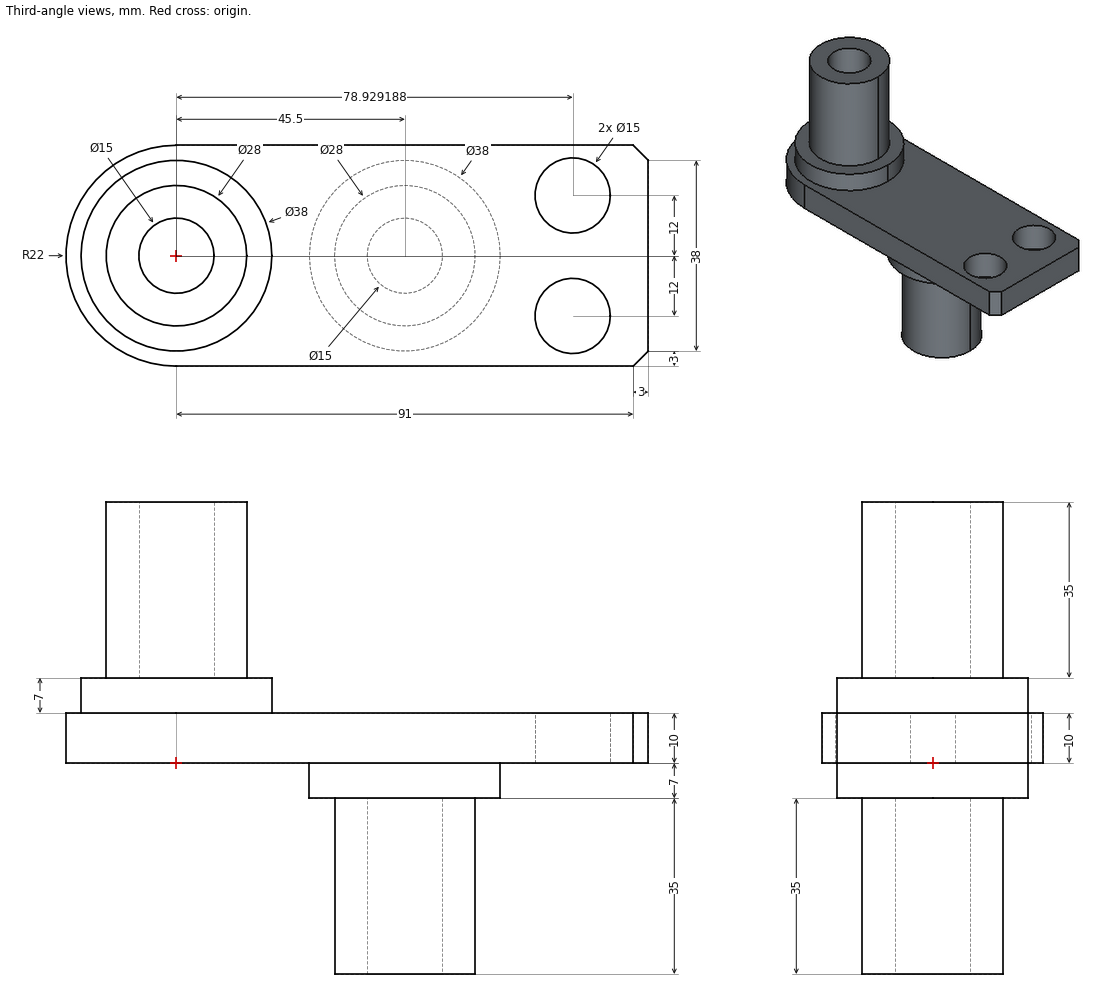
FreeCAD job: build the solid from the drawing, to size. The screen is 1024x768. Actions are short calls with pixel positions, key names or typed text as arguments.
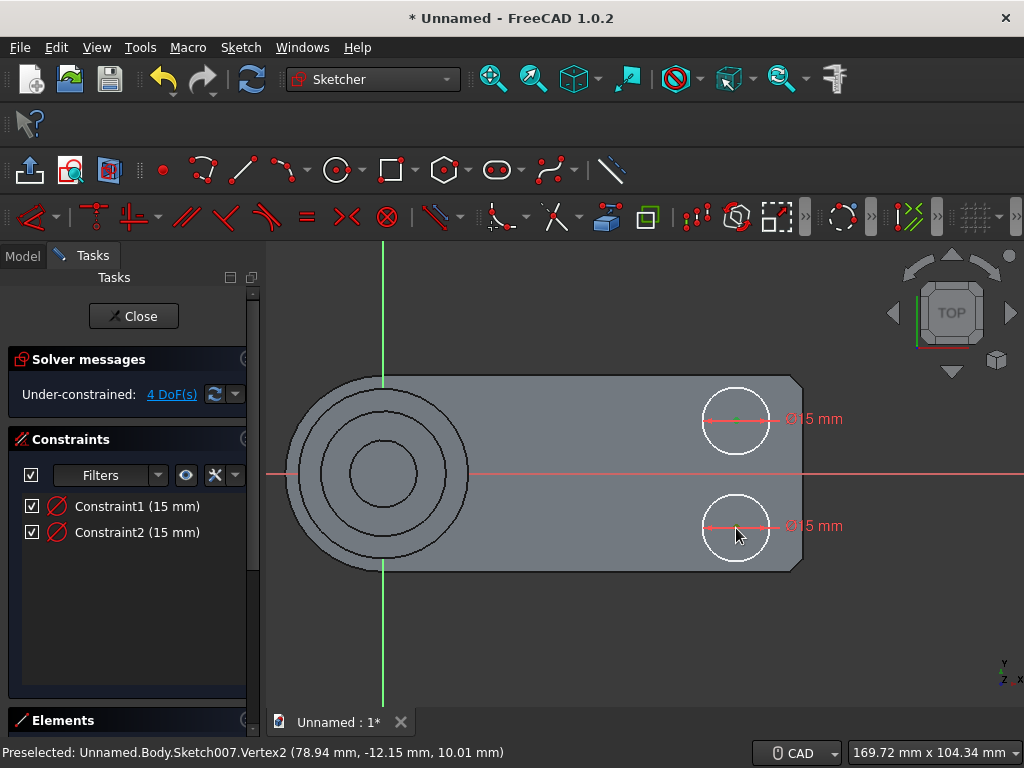
click(160, 218)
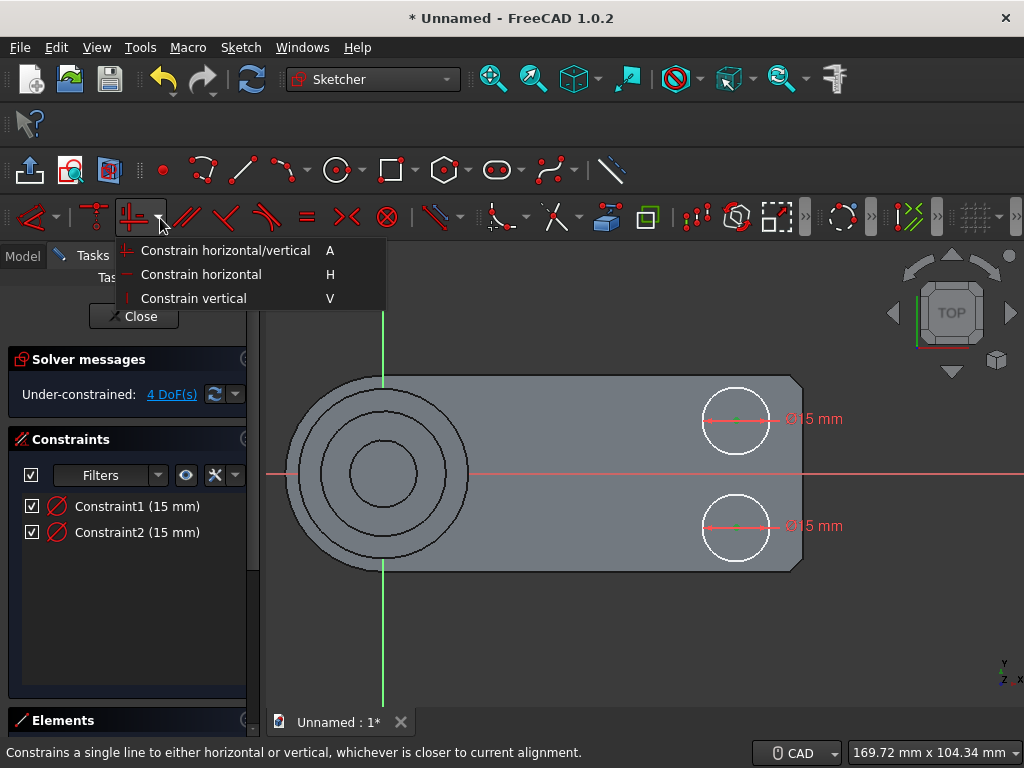
click(251, 298)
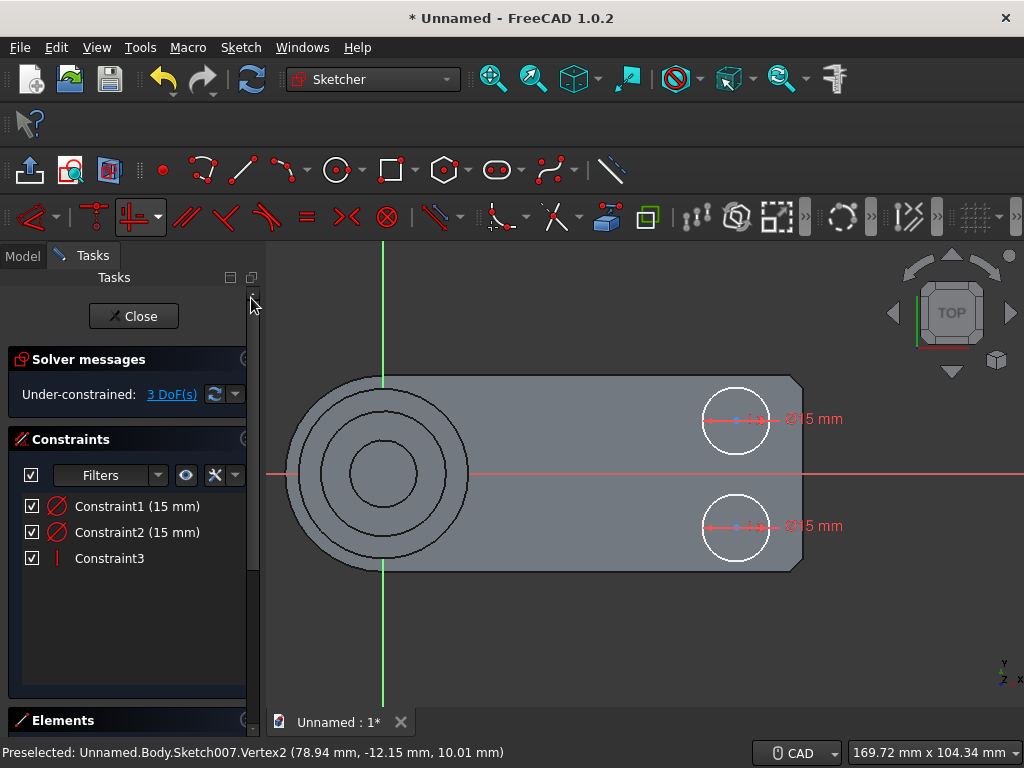
click(32, 218)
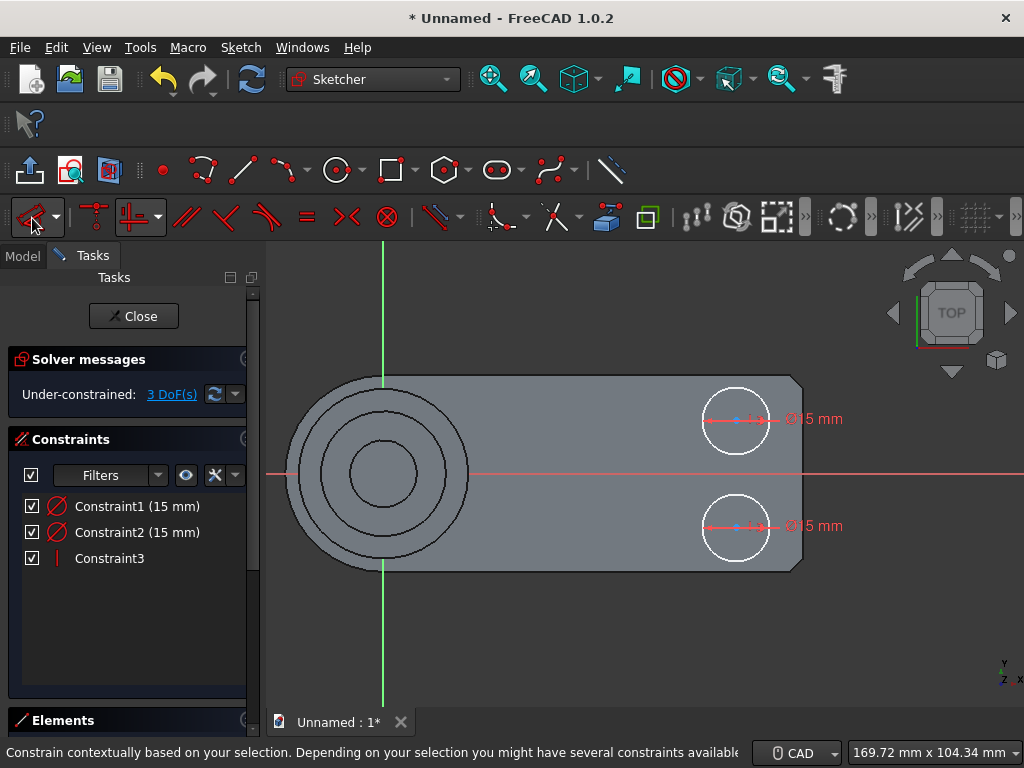
click(736, 421)
click(349, 447)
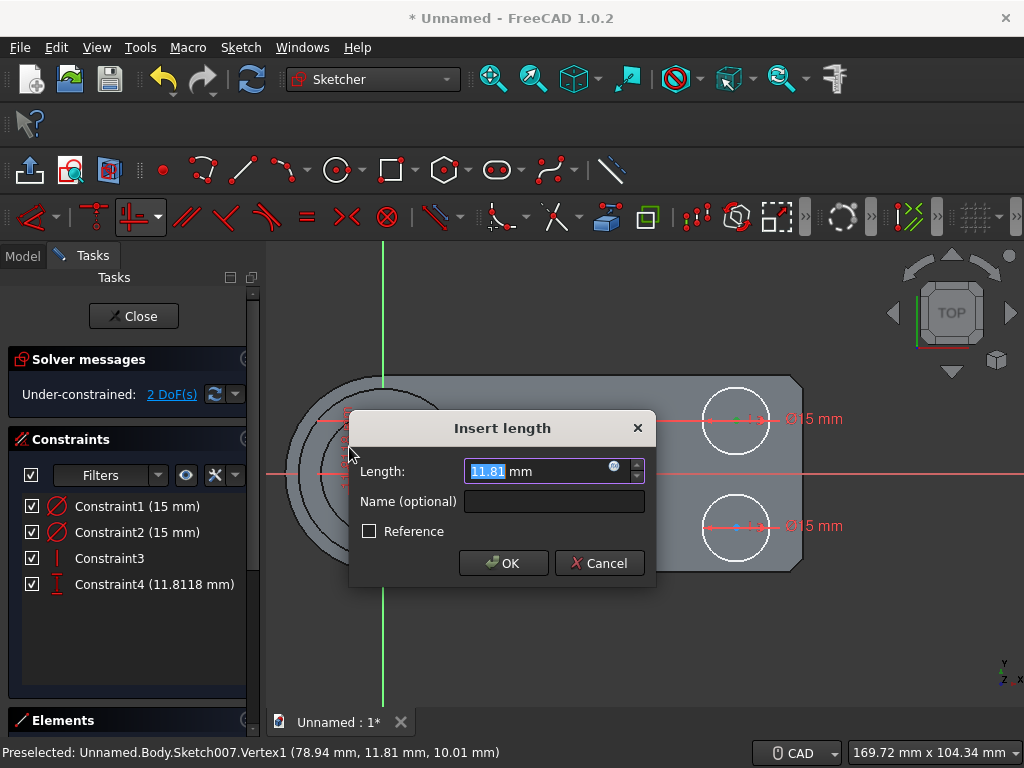
text(12)
key(Return)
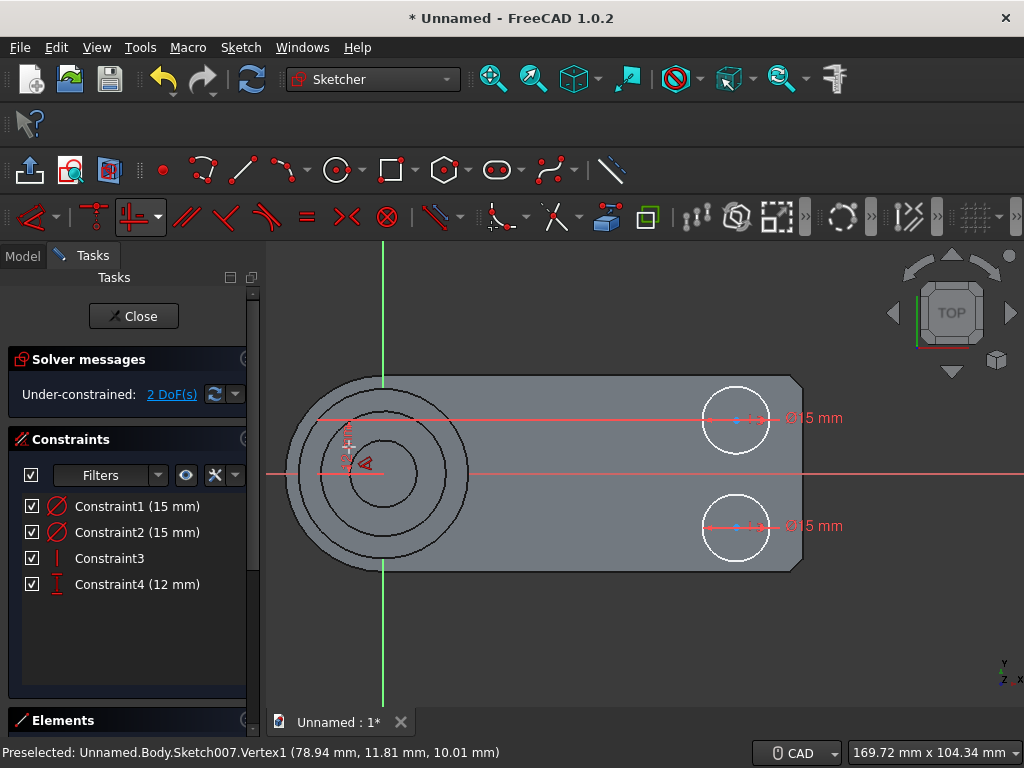
click(736, 528)
click(349, 501)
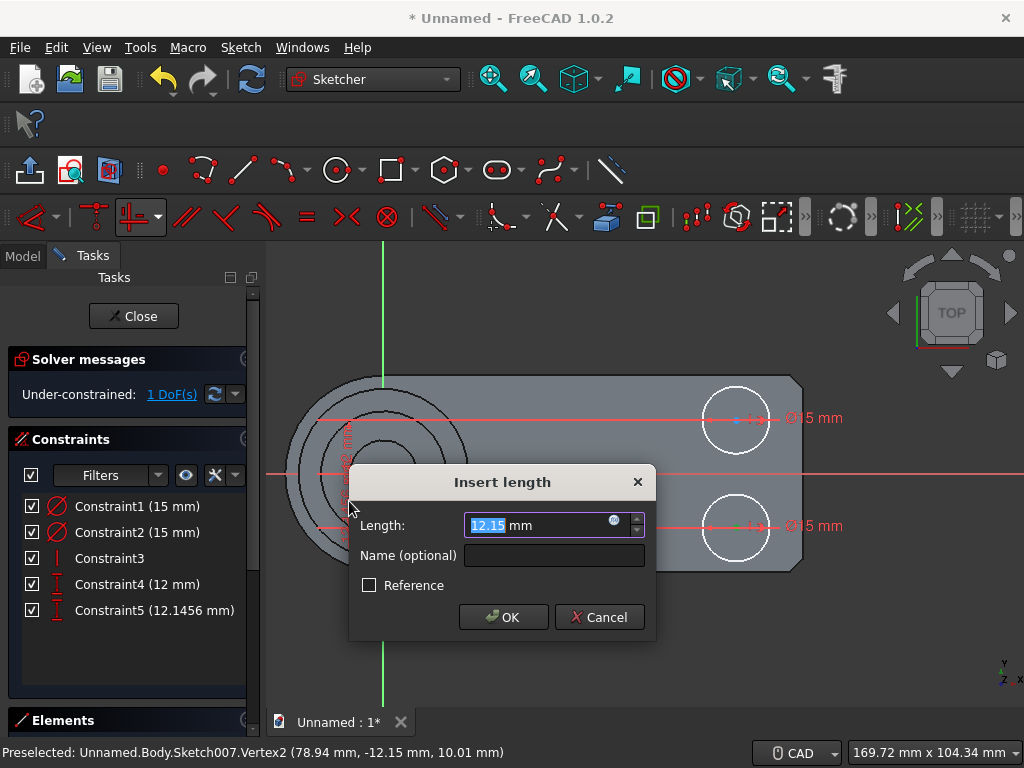
text(12)
key(Return)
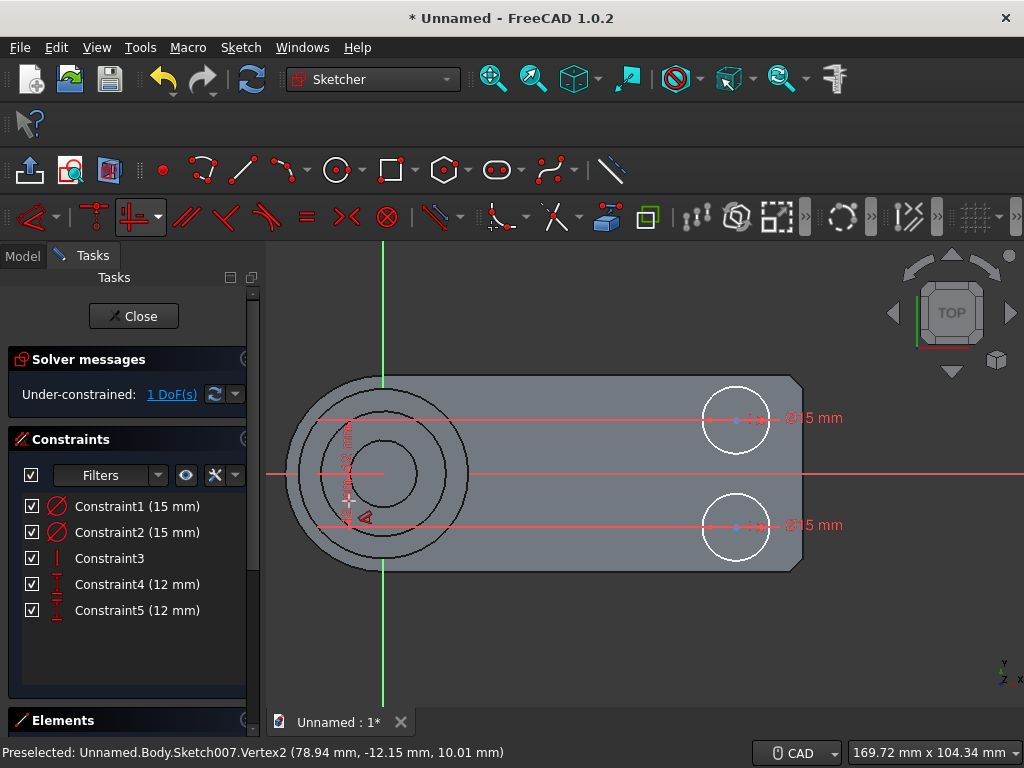
click(736, 420)
click(560, 386)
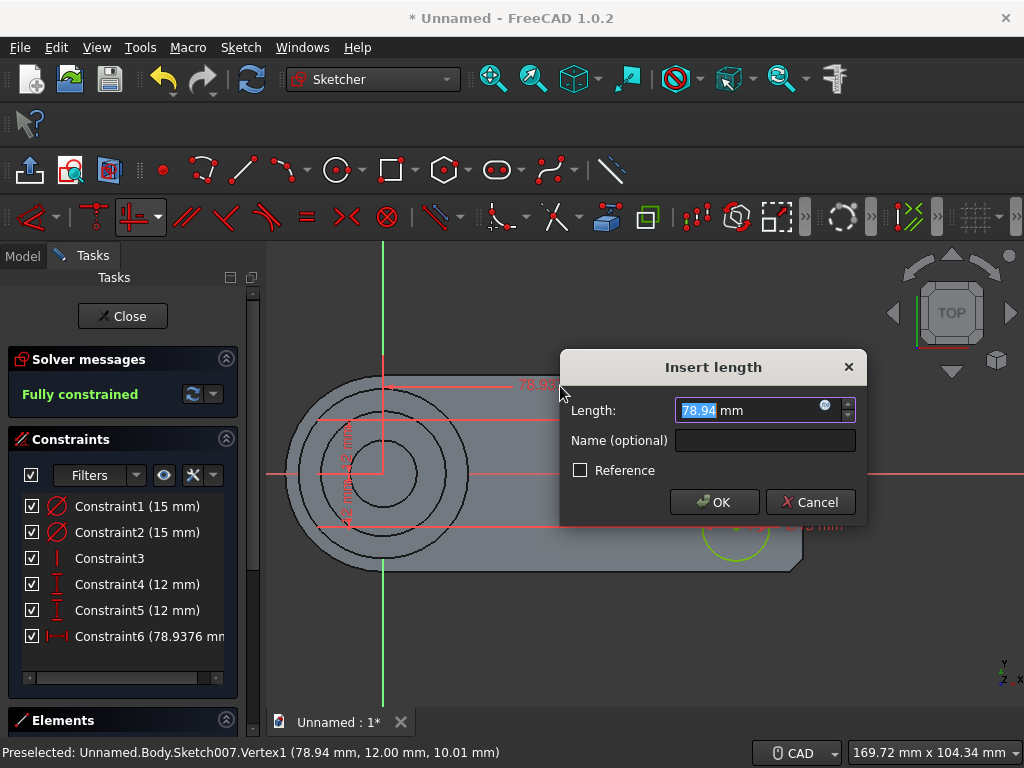
text(78.929188)
key(Return)
key(Escape)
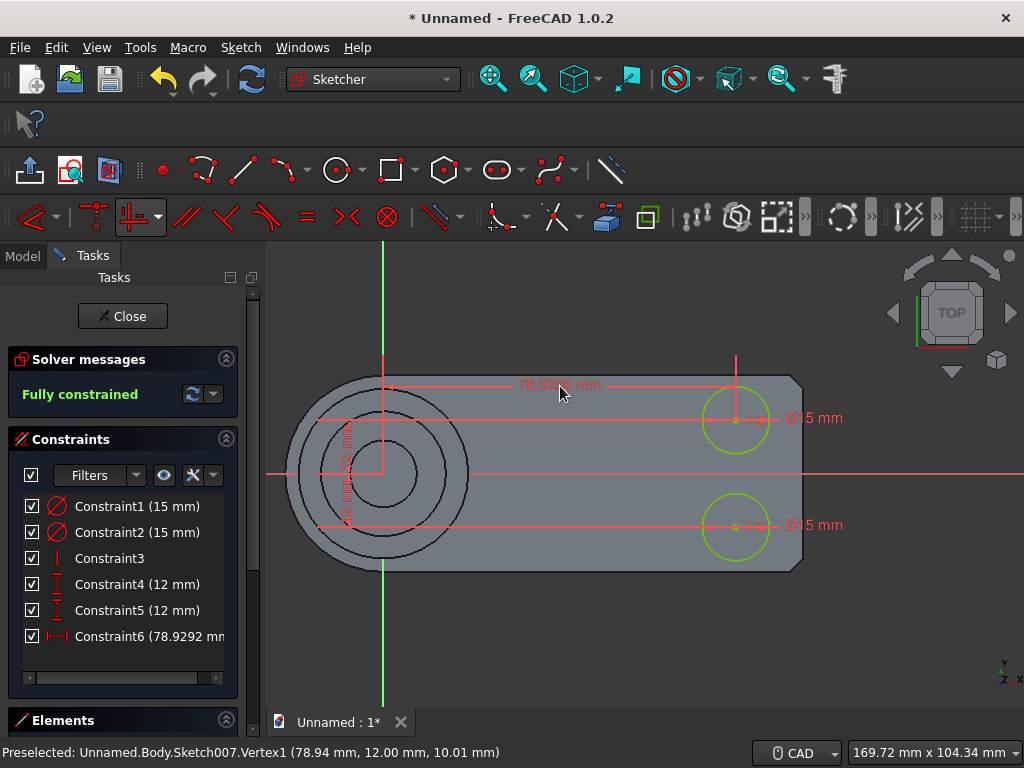
click(123, 316)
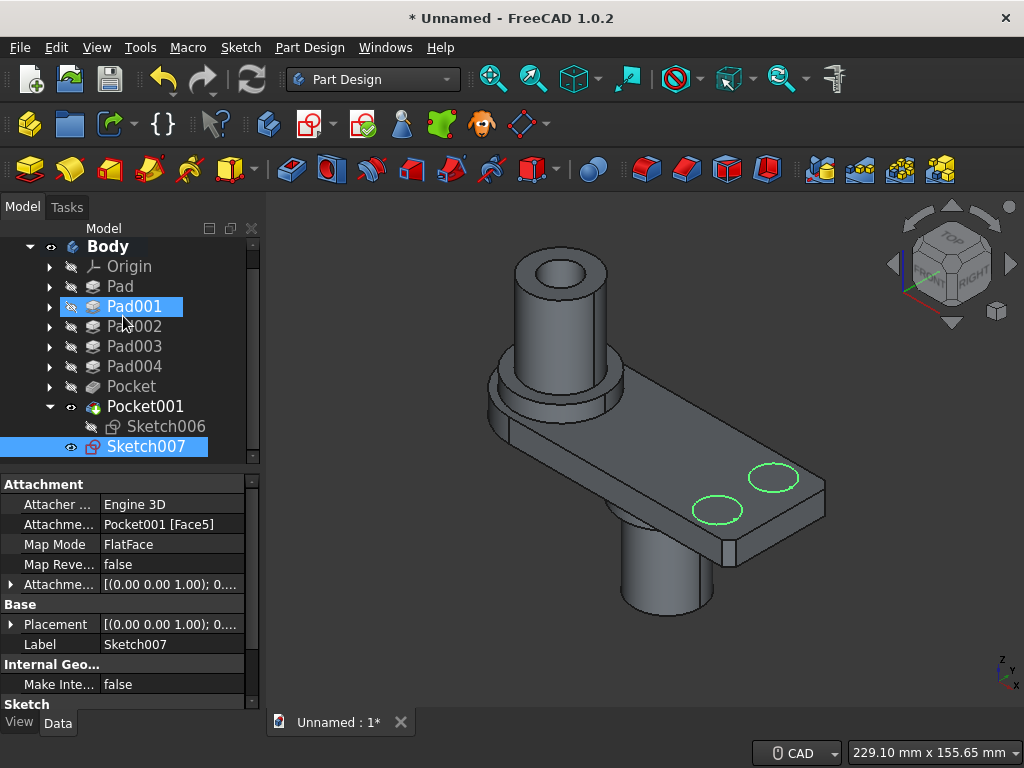
click(292, 170)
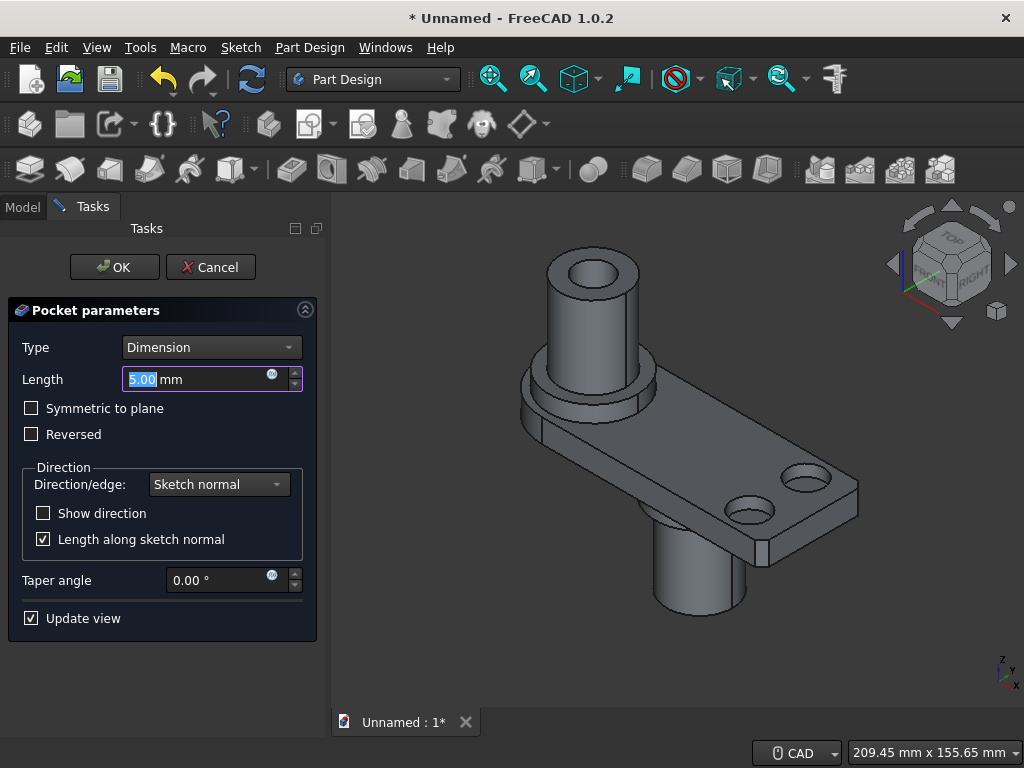
text(10)
key(Tab)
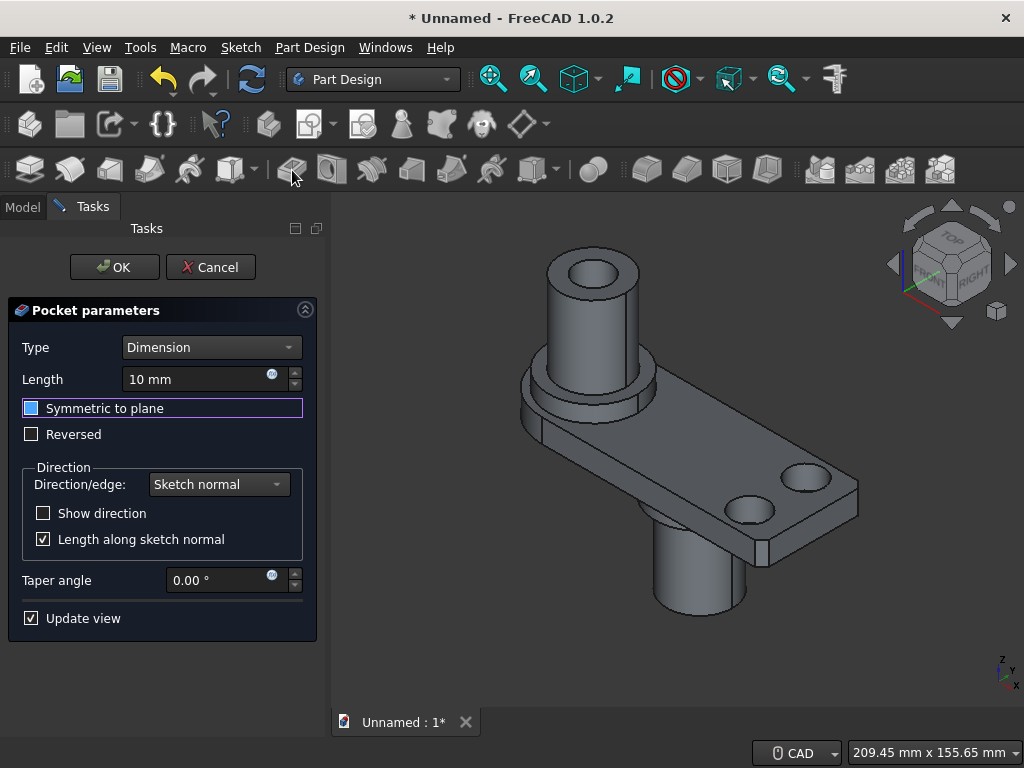
click(115, 267)